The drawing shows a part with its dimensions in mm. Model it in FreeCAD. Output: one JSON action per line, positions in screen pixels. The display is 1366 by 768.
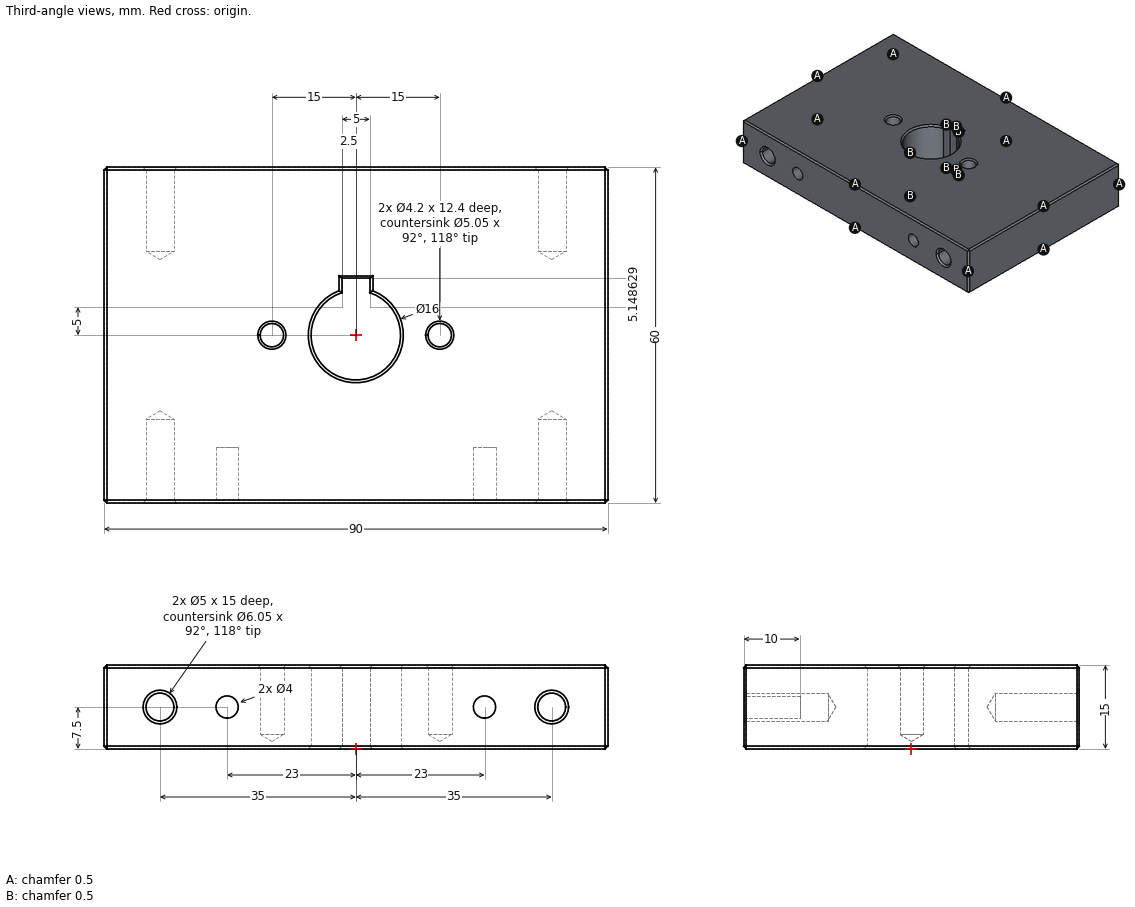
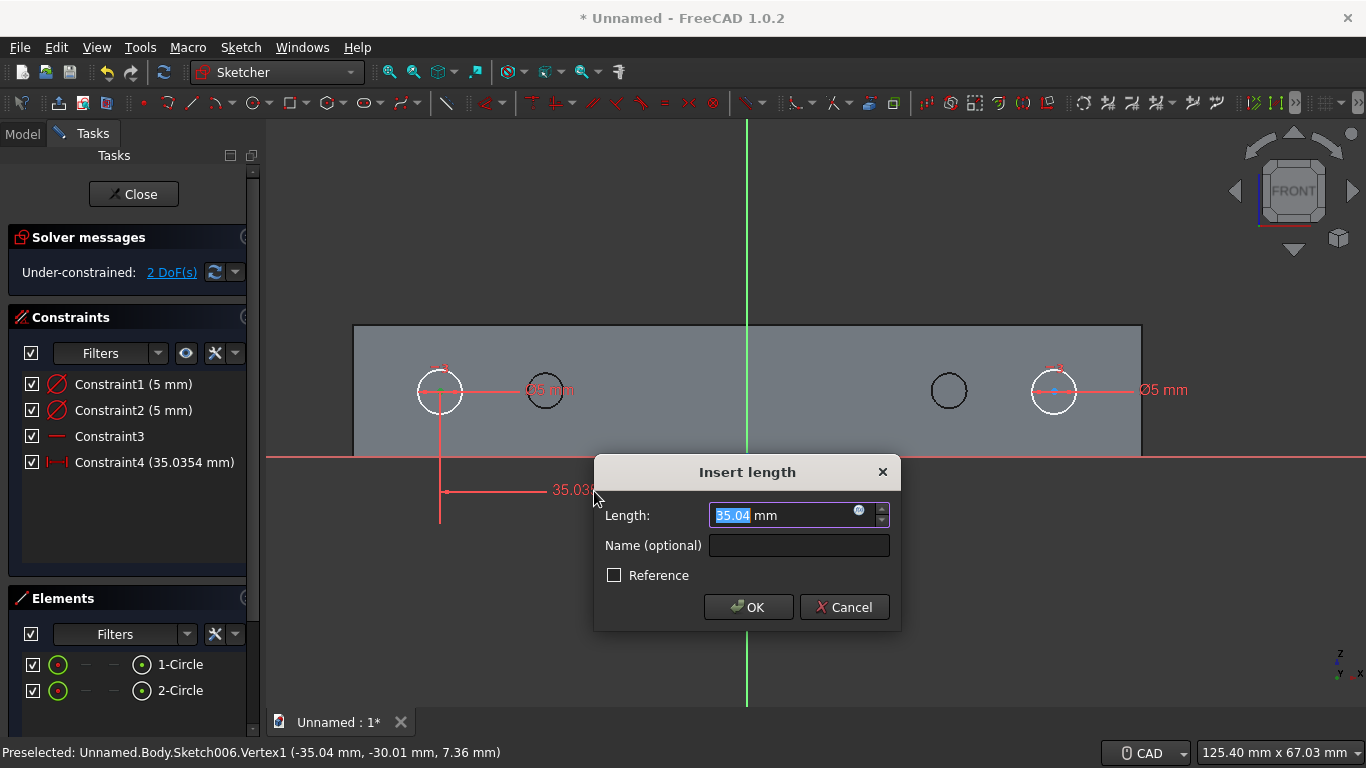
{"action": "type", "text": "35"}
{"action": "key", "text": "Return"}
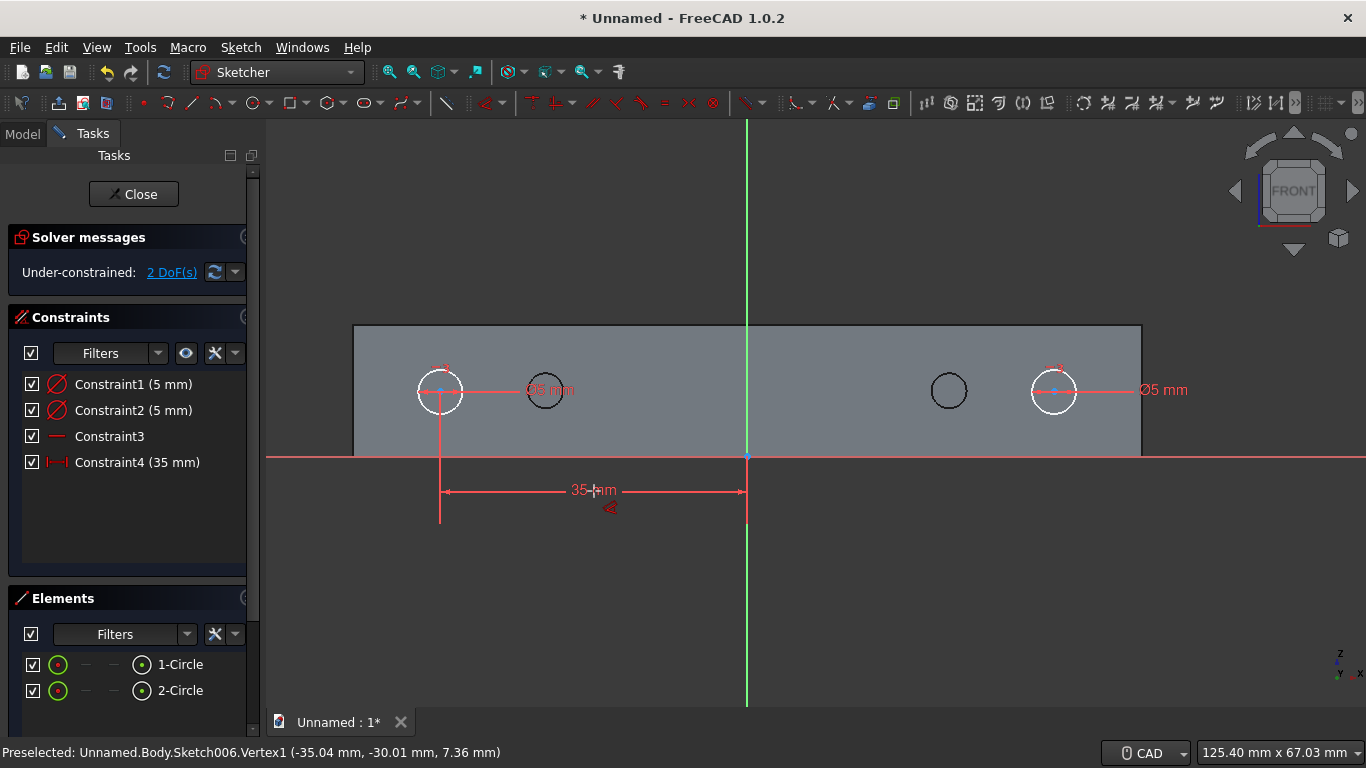
{"action": "left_click", "coordinate": [1054, 392]}
{"action": "left_click", "coordinate": [901, 491]}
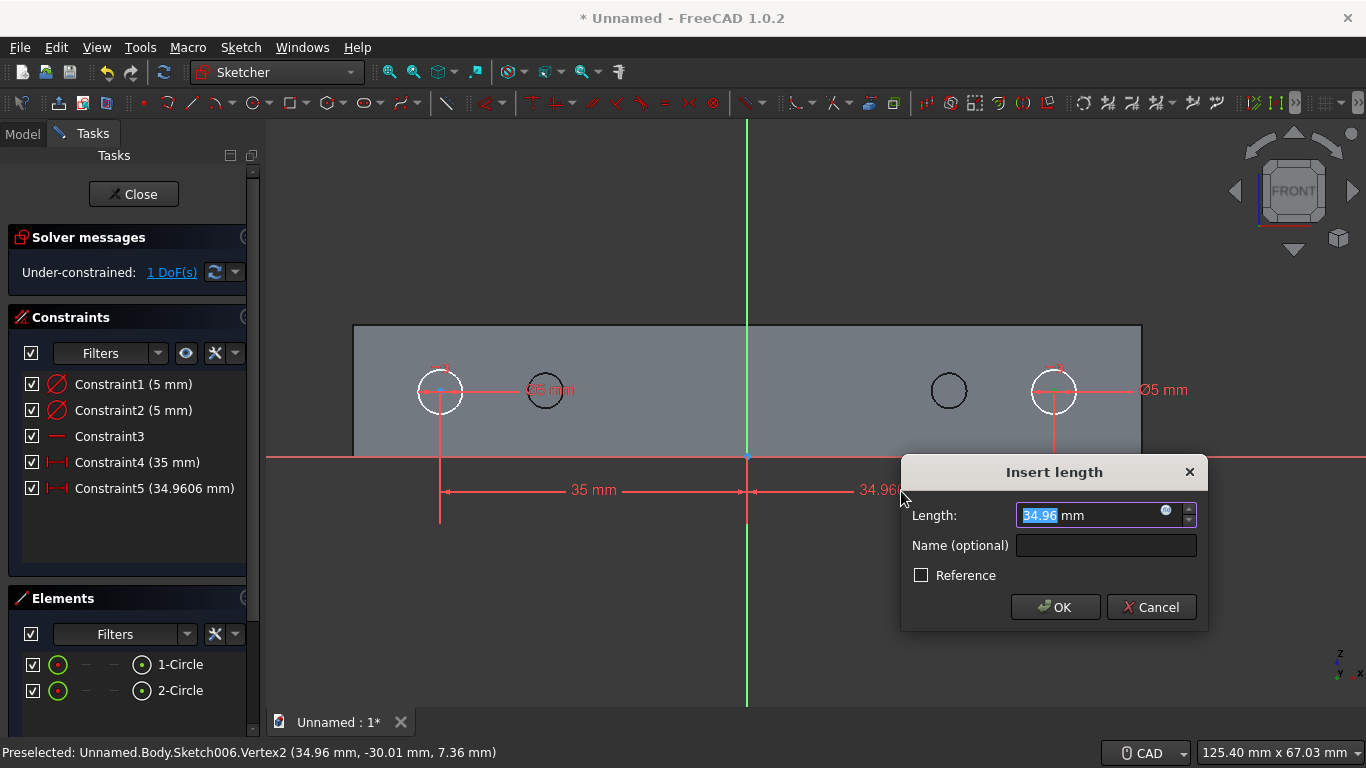
{"action": "type", "text": "35"}
{"action": "key", "text": "Return"}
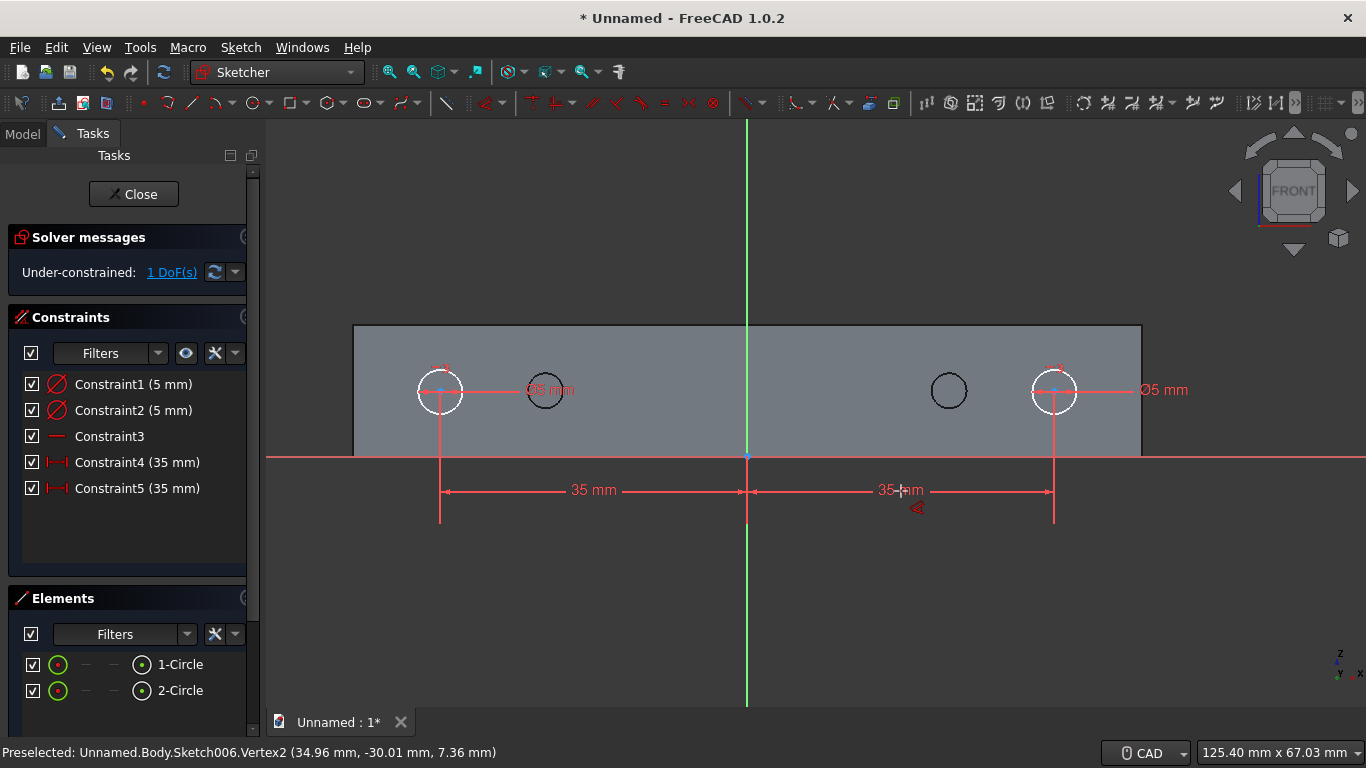
{"action": "left_click", "coordinate": [440, 392]}
{"action": "left_click", "coordinate": [406, 424]}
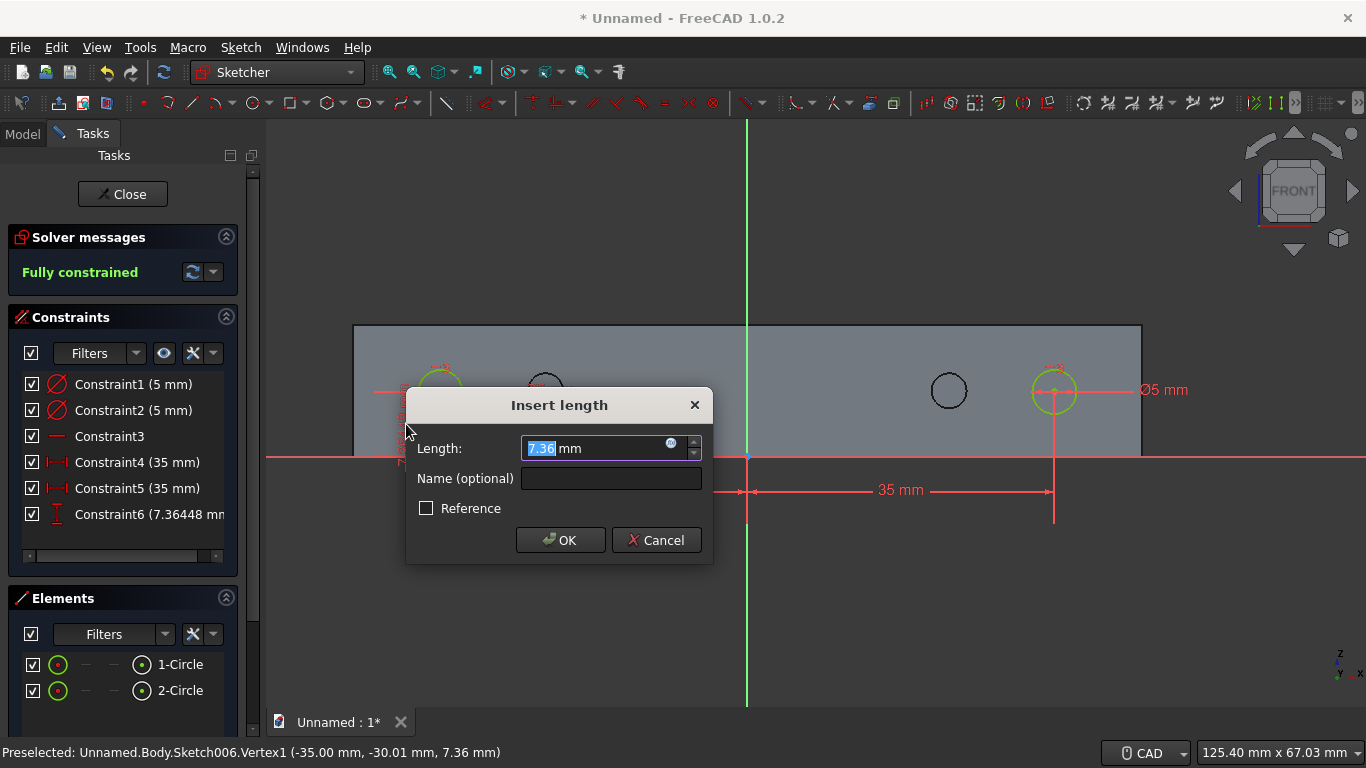
{"action": "type", "text": "7.5"}
{"action": "key", "text": "Return"}
{"action": "key", "text": "Escape"}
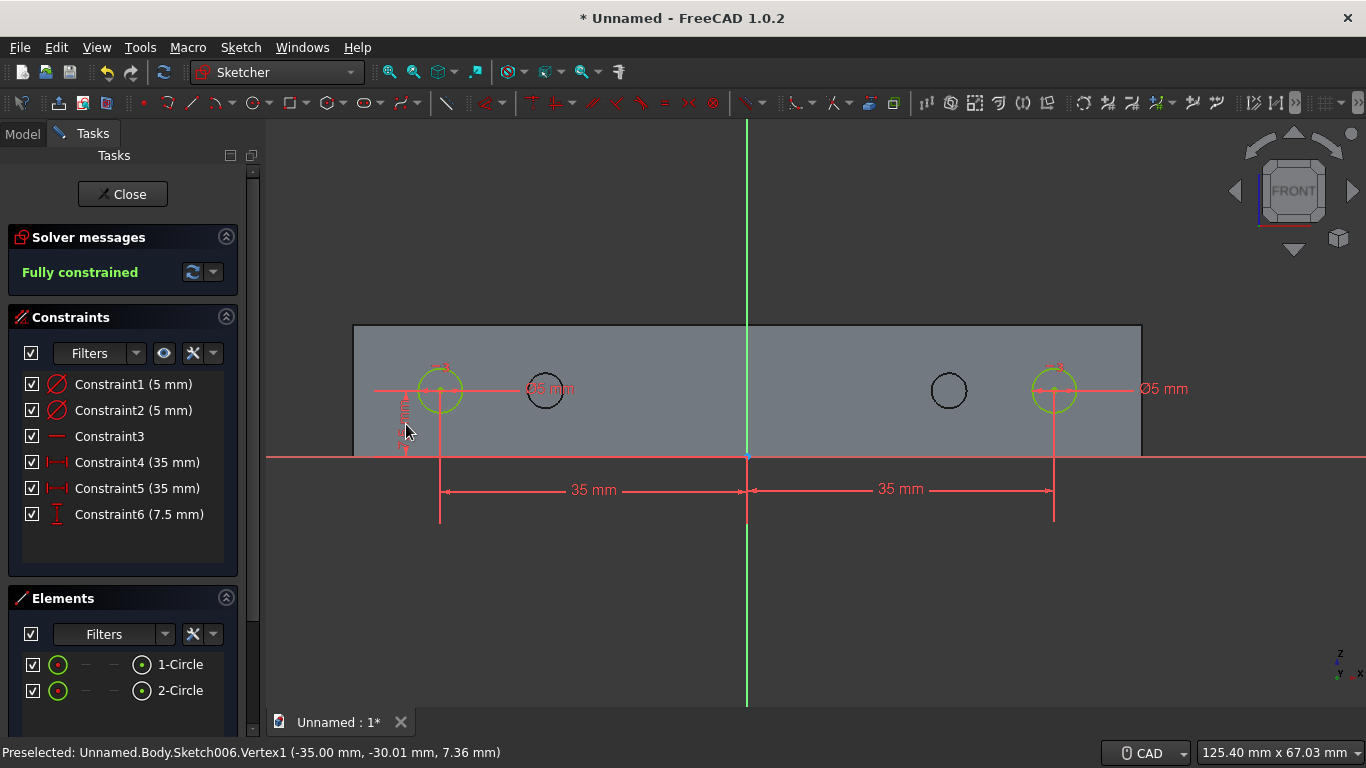
{"action": "left_click", "coordinate": [123, 194]}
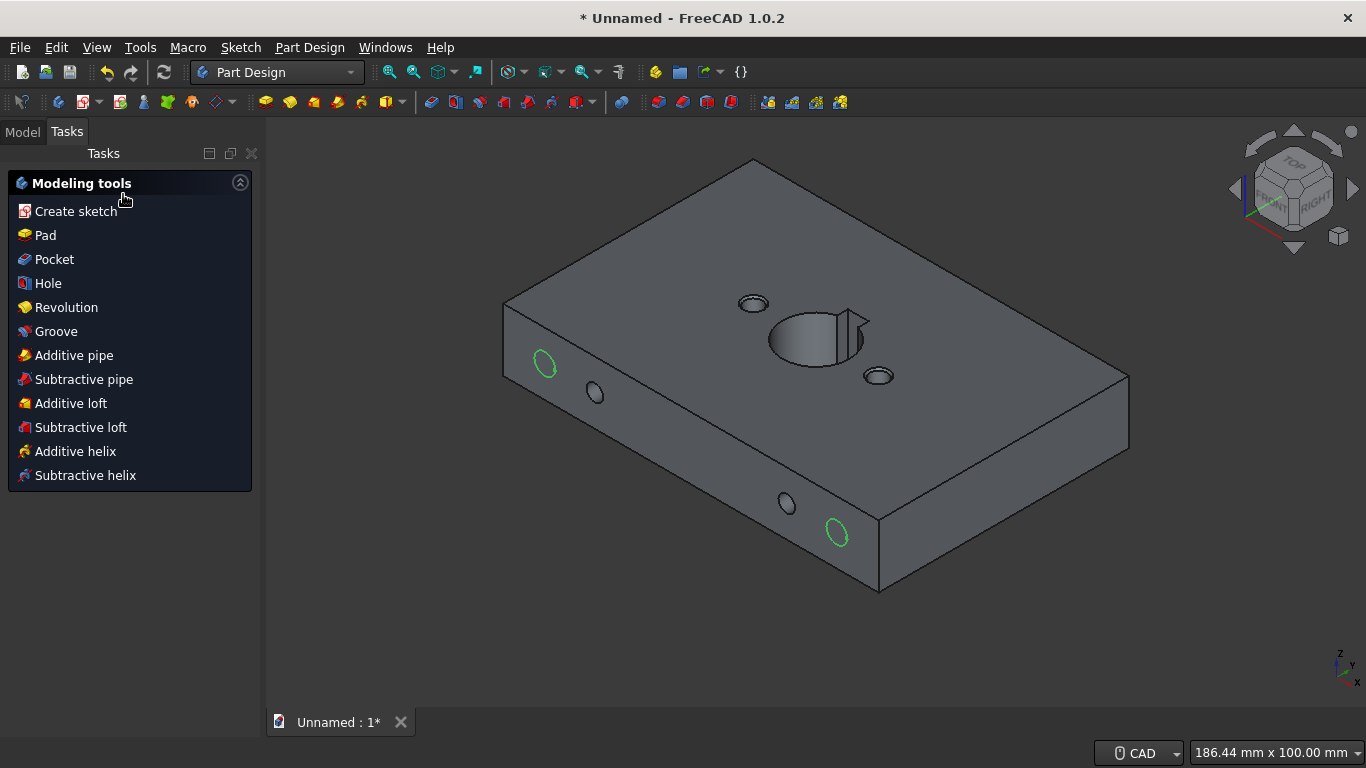
{"action": "left_click", "coordinate": [456, 102]}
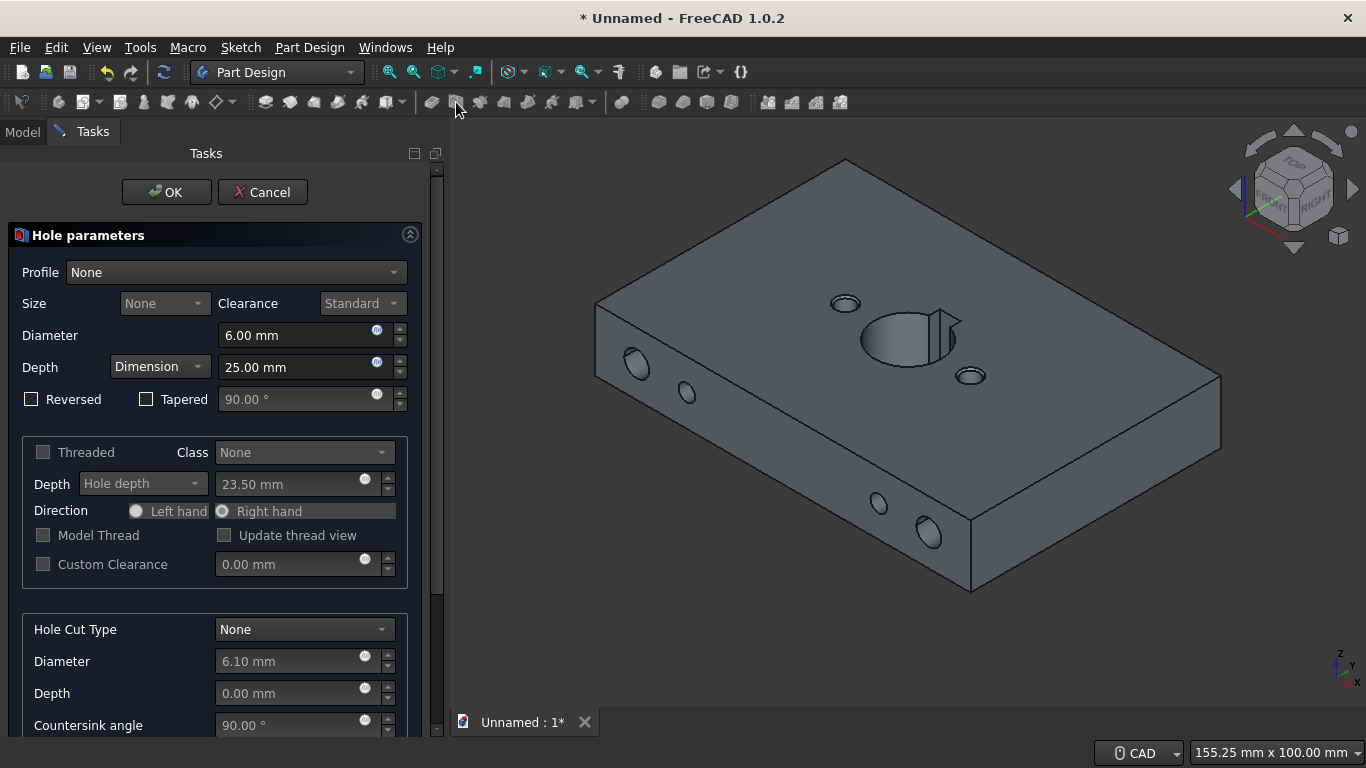
{"action": "triple_click", "coordinate": [305, 335]}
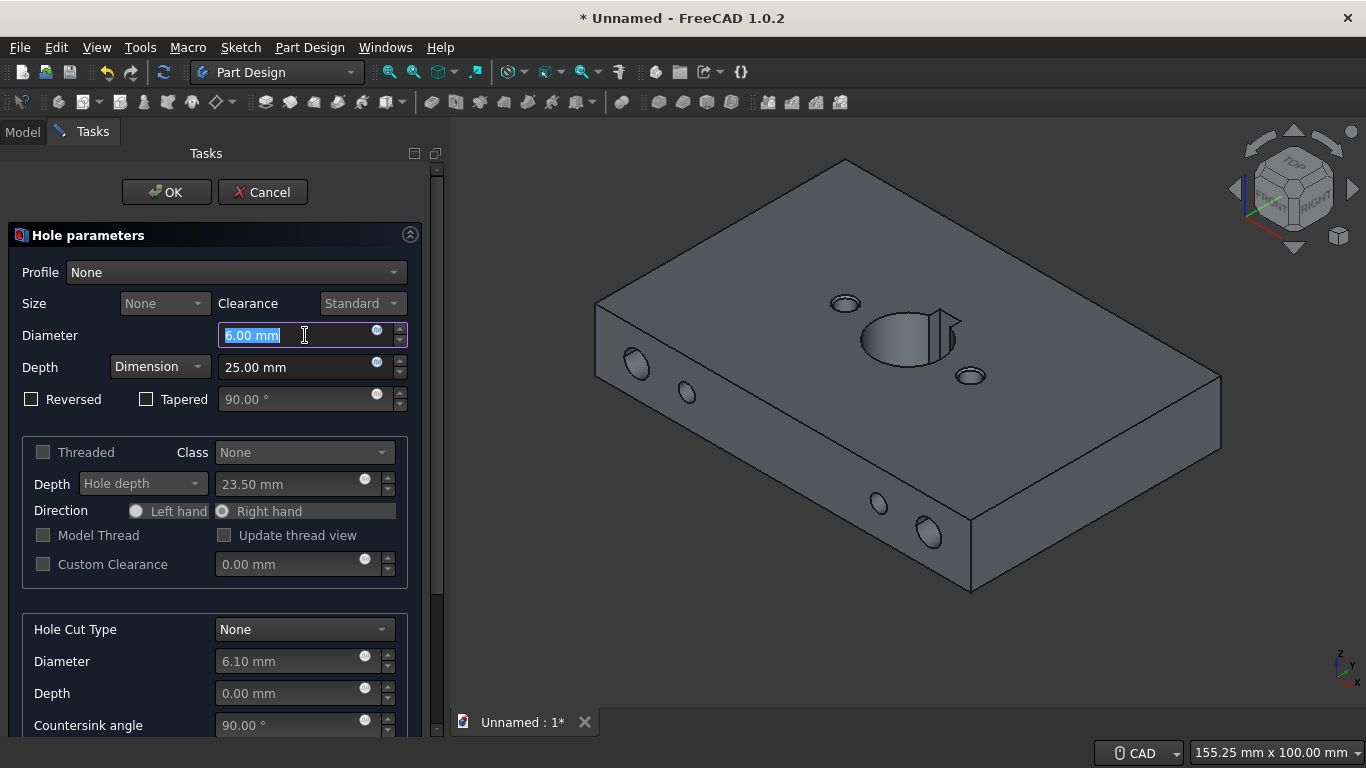
{"action": "type", "text": "5"}
{"action": "key", "text": "Tab"}